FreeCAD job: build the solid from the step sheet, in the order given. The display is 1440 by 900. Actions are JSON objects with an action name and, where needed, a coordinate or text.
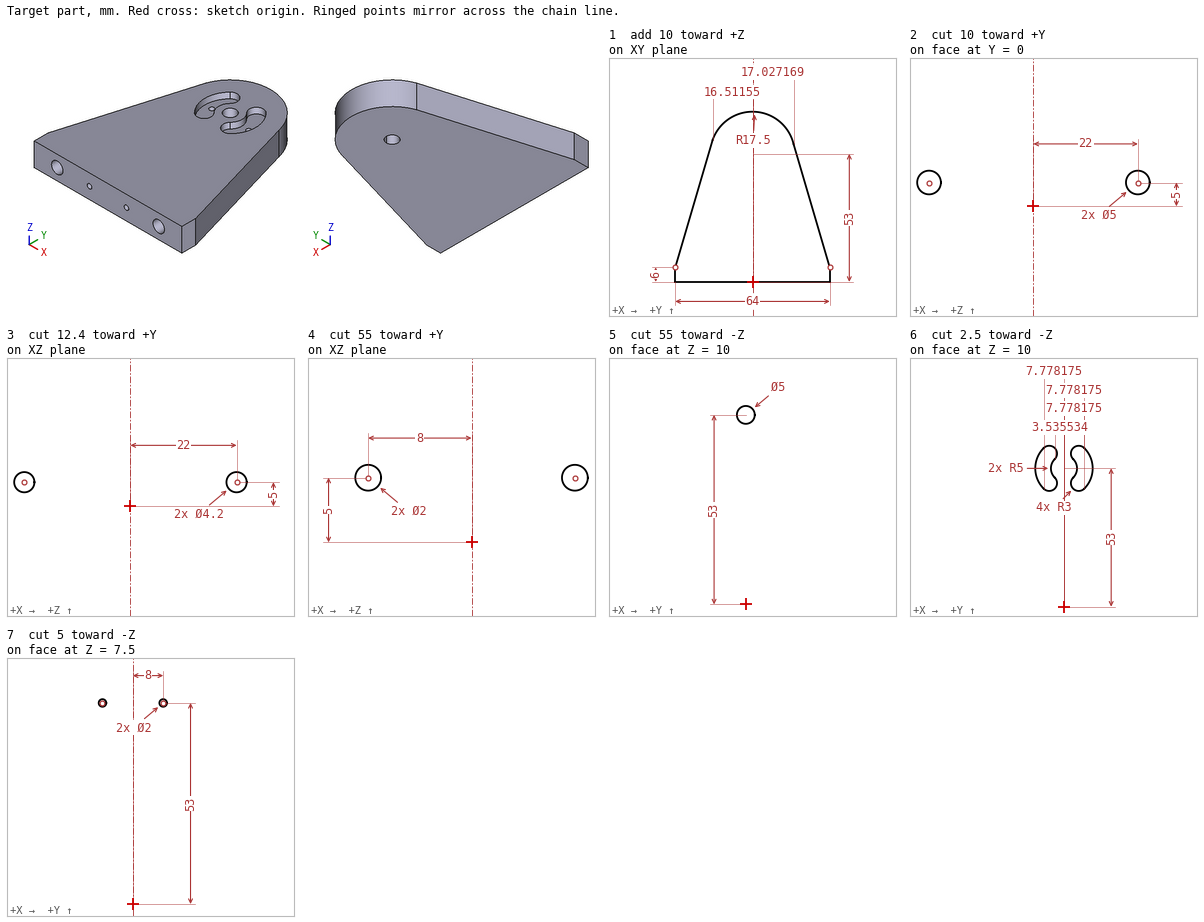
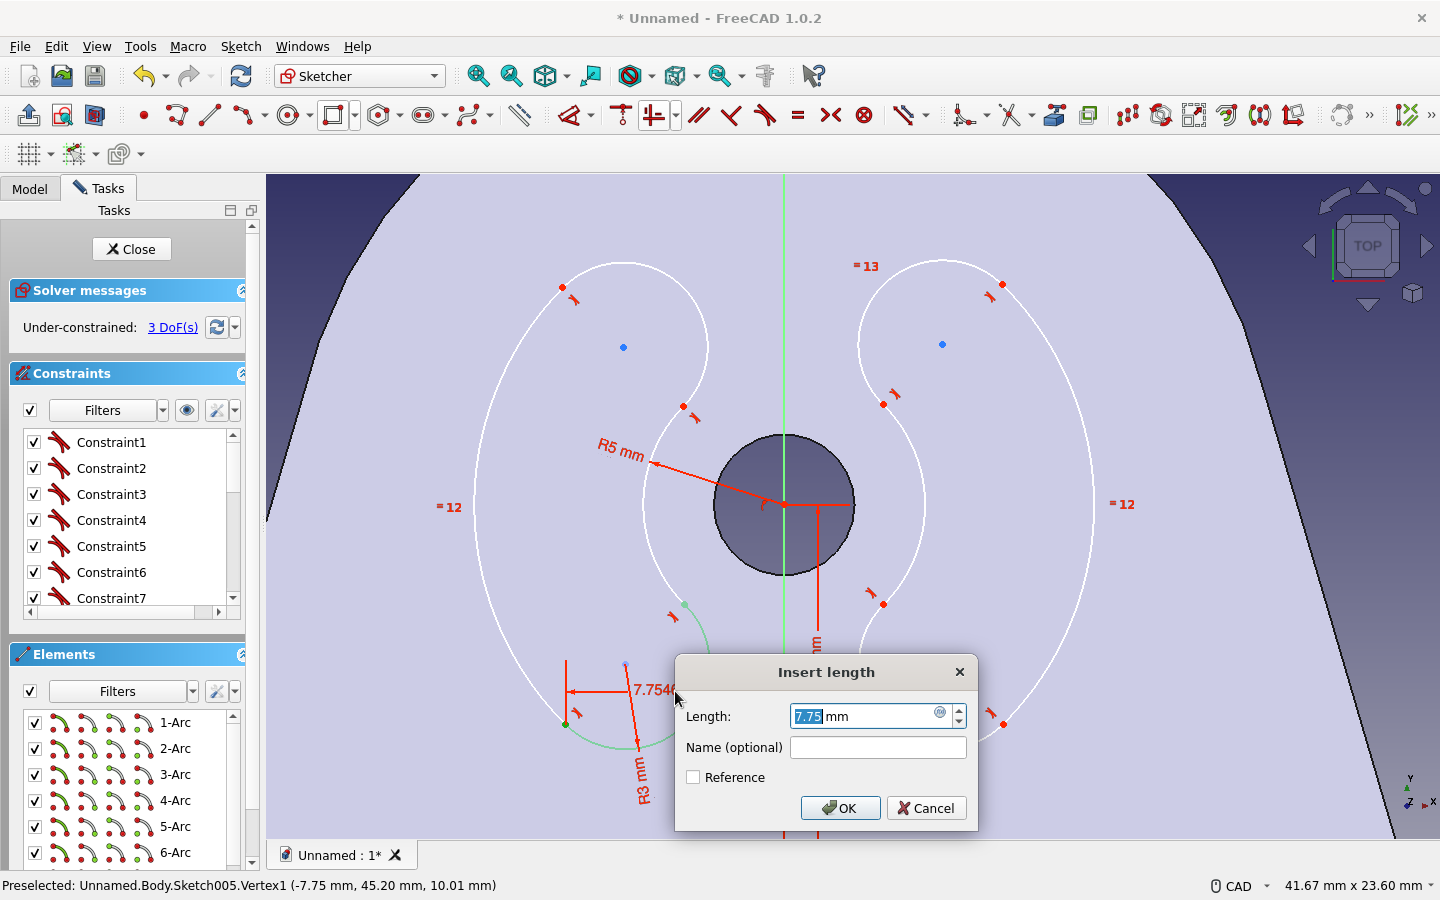
{"action": "type", "text": "7.778175"}
{"action": "key", "text": "Return"}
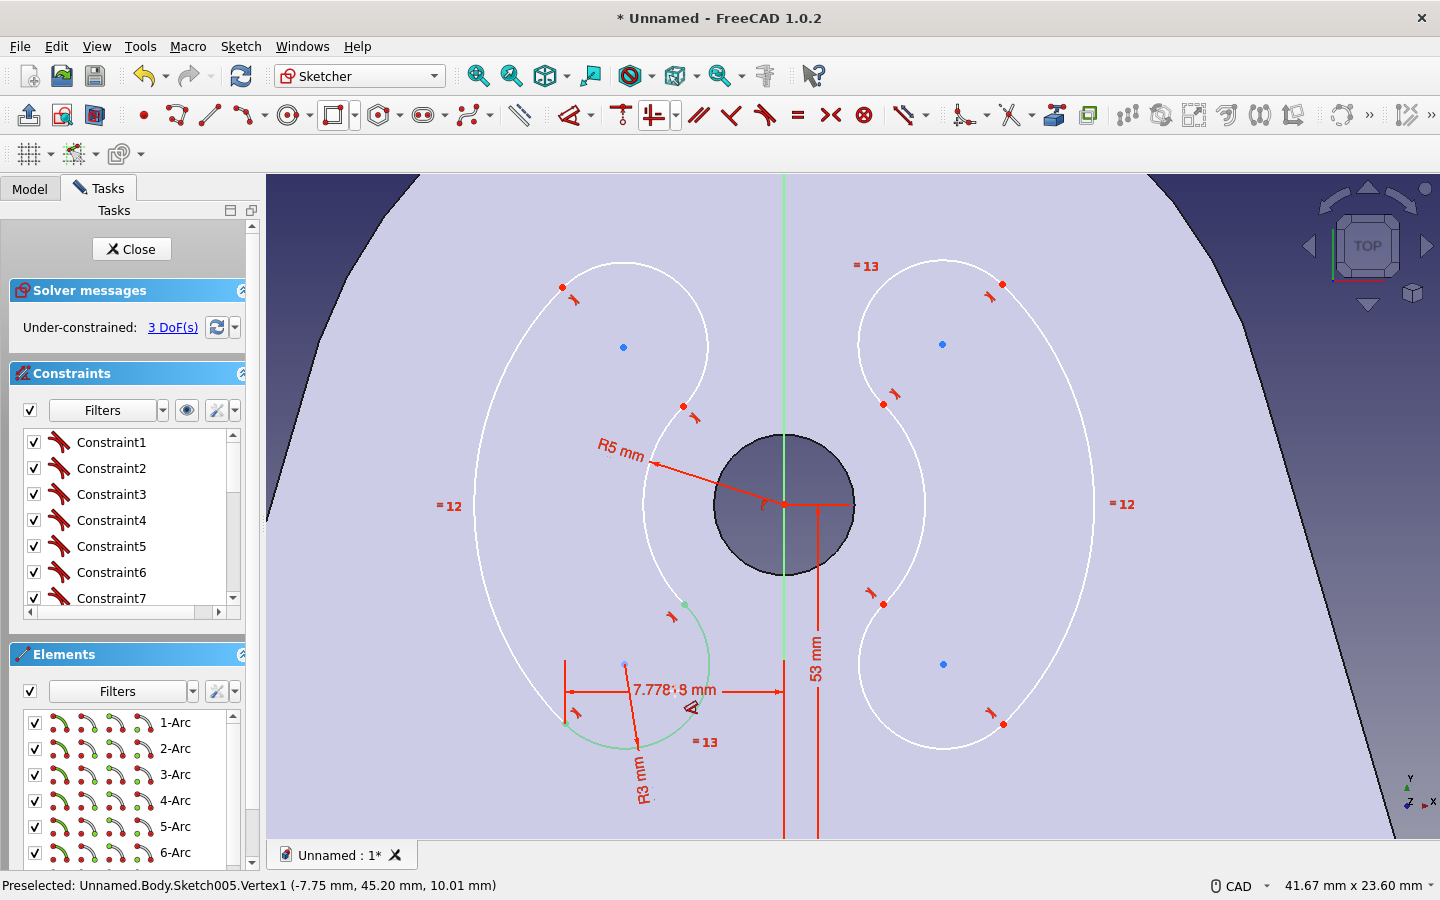
{"action": "left_click", "coordinate": [684, 406]}
{"action": "left_click", "coordinate": [734, 372]}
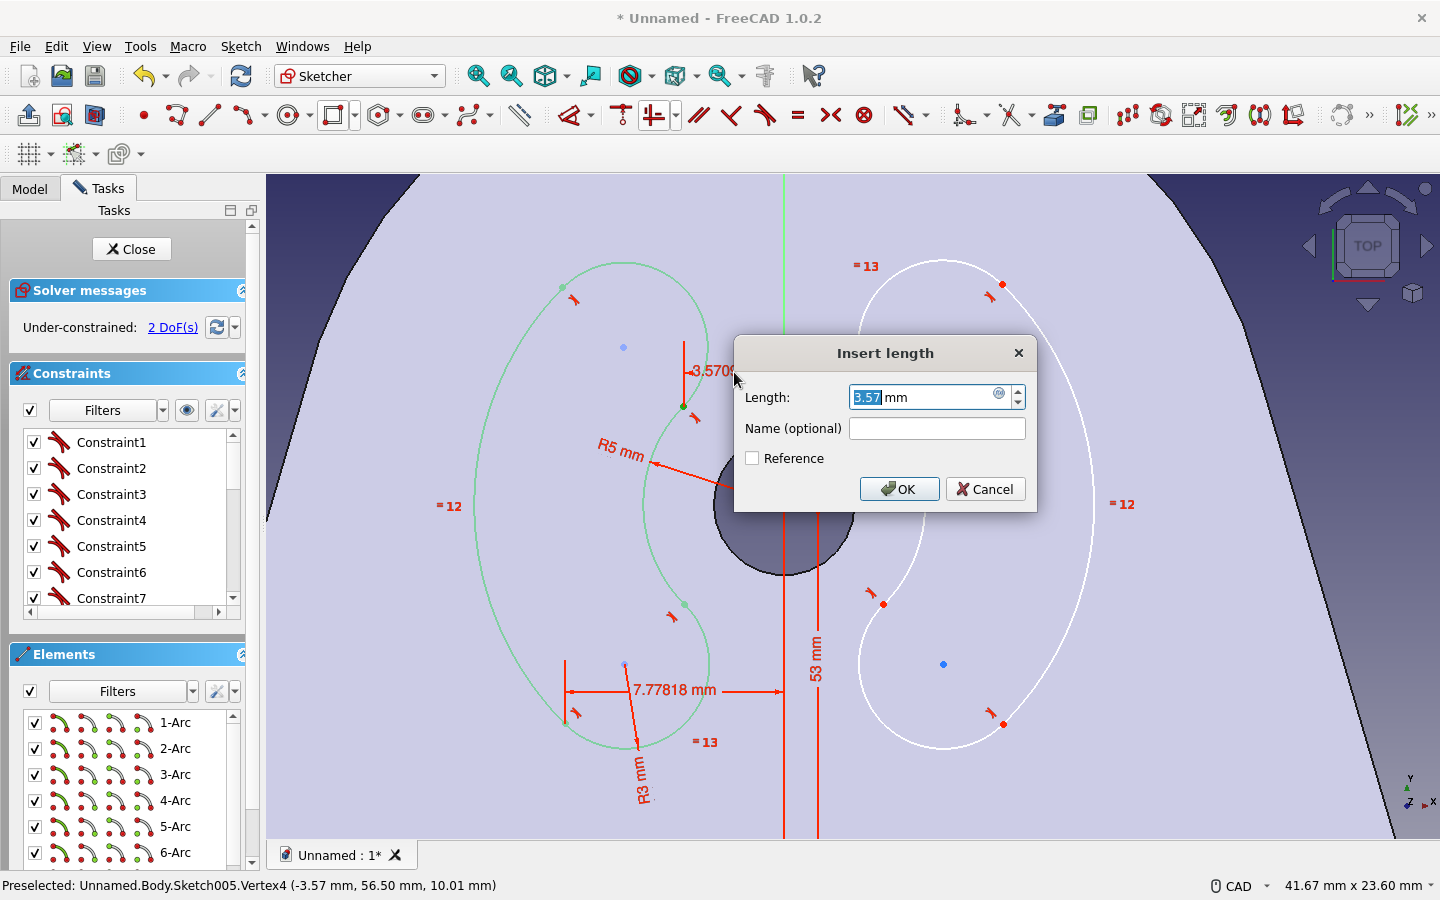
{"action": "type", "text": "3.535534"}
{"action": "key", "text": "Return"}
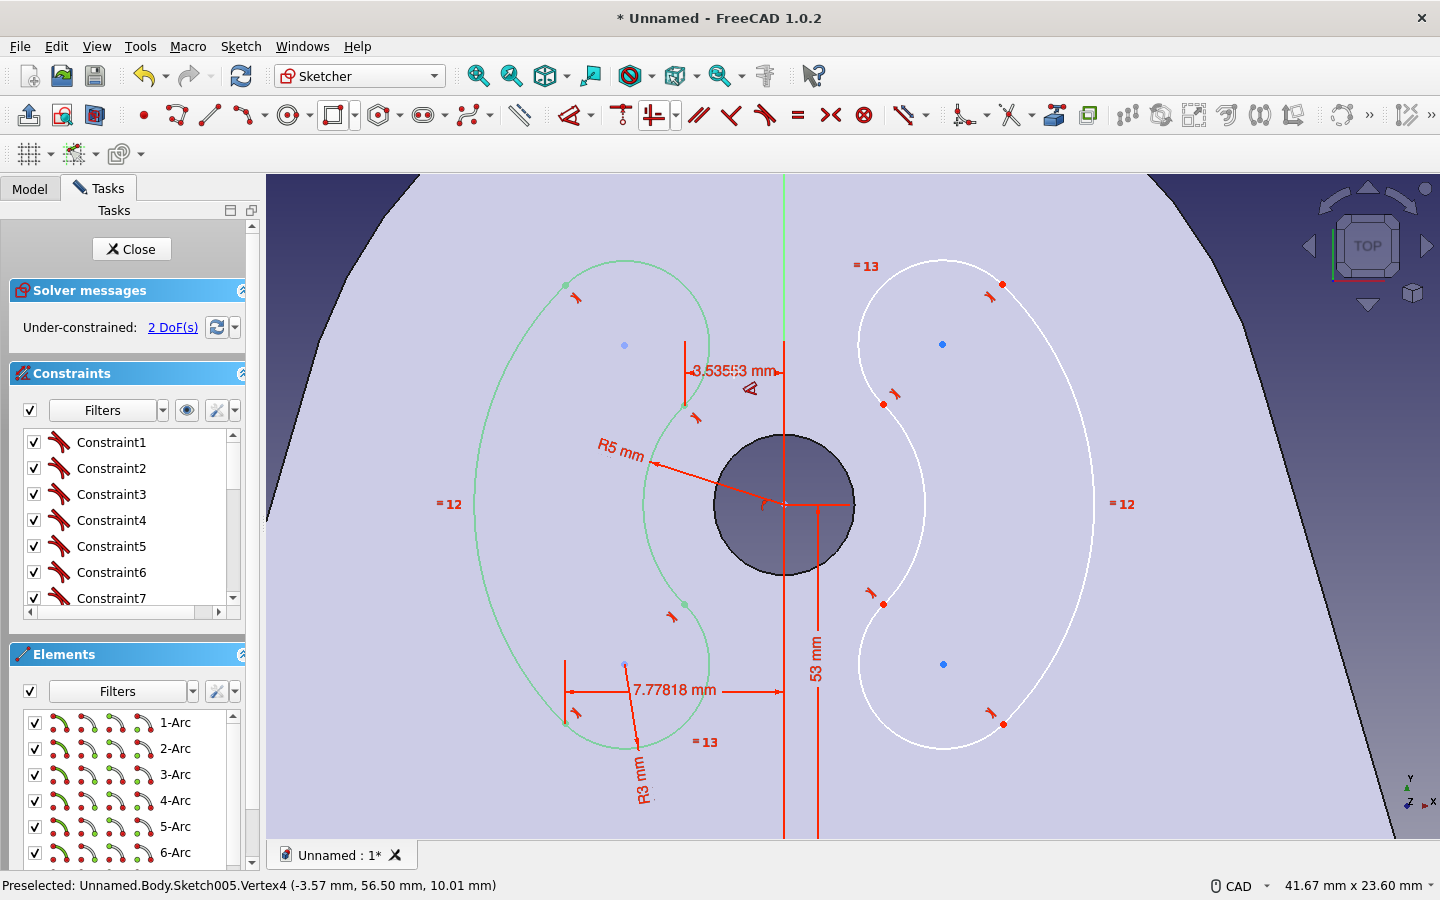
{"action": "left_click", "coordinate": [1003, 724]}
{"action": "left_click", "coordinate": [894, 690]}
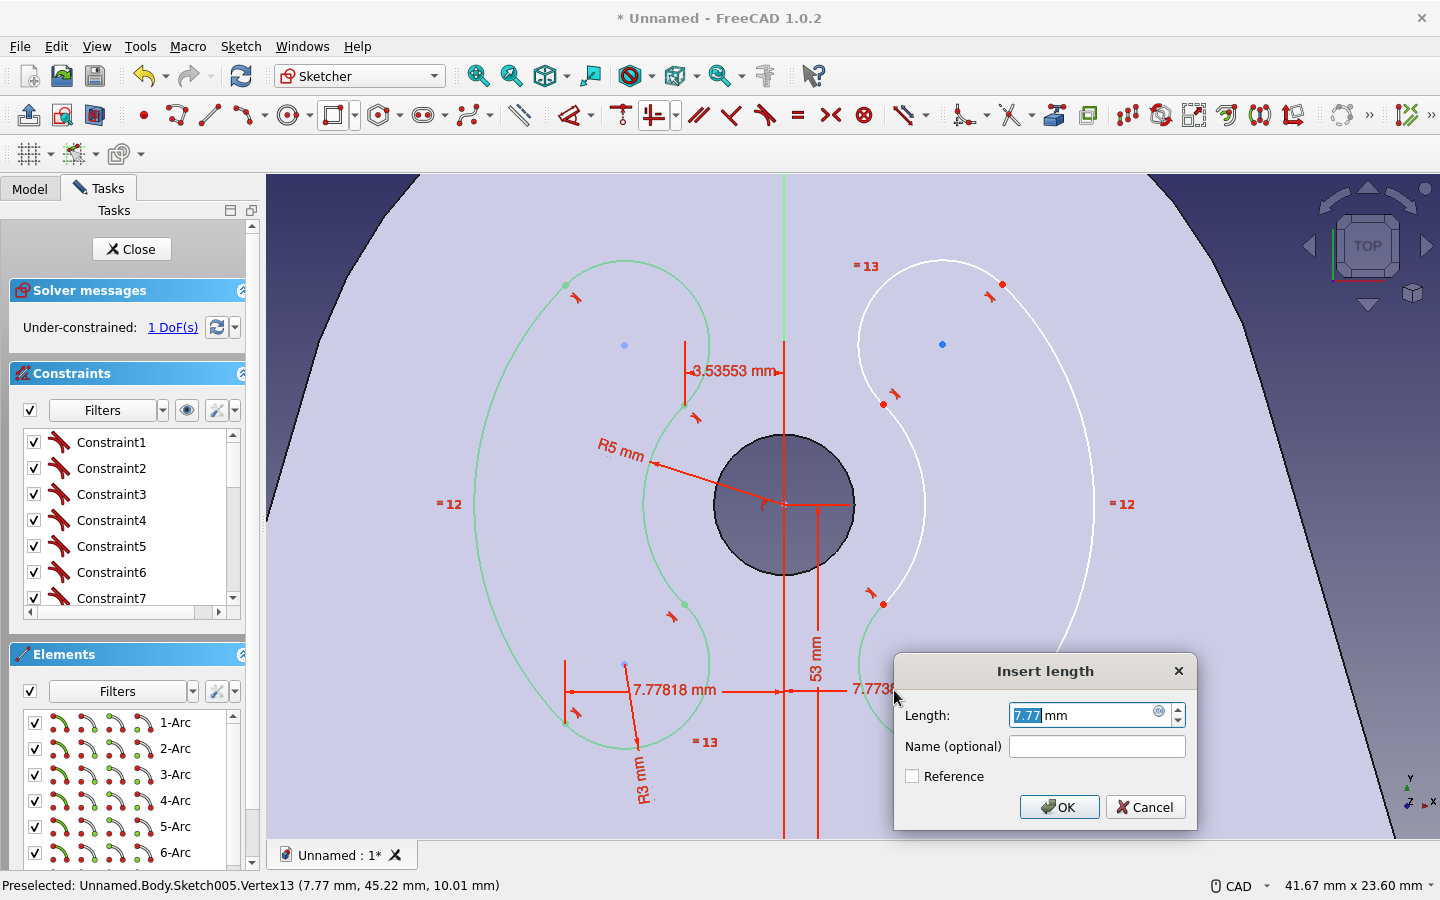
{"action": "type", "text": "7.778175"}
{"action": "key", "text": "Return"}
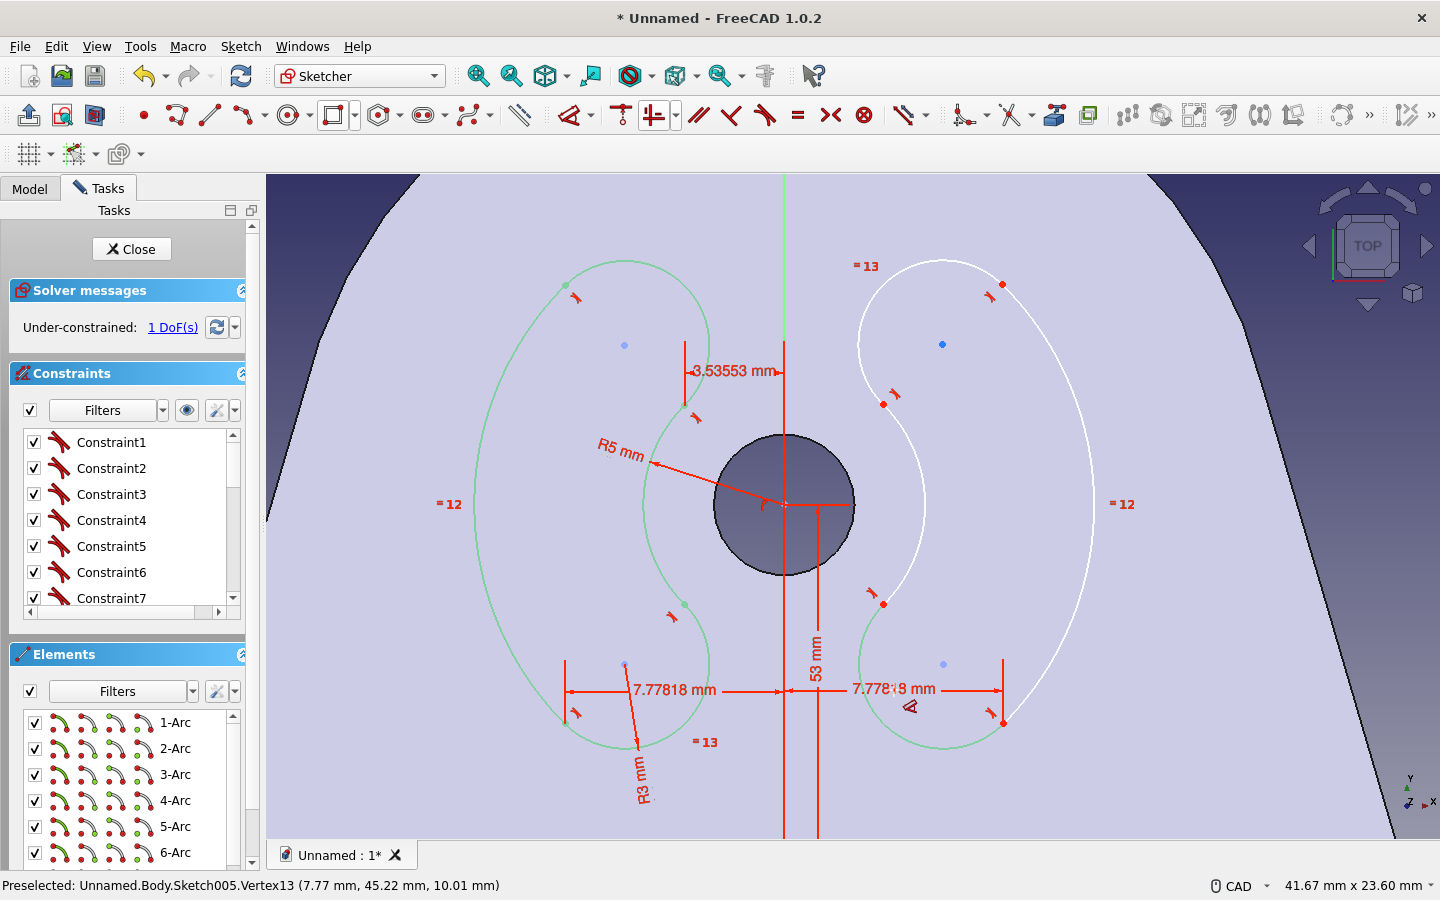
{"action": "left_click", "coordinate": [1002, 285]}
{"action": "left_click", "coordinate": [893, 251]}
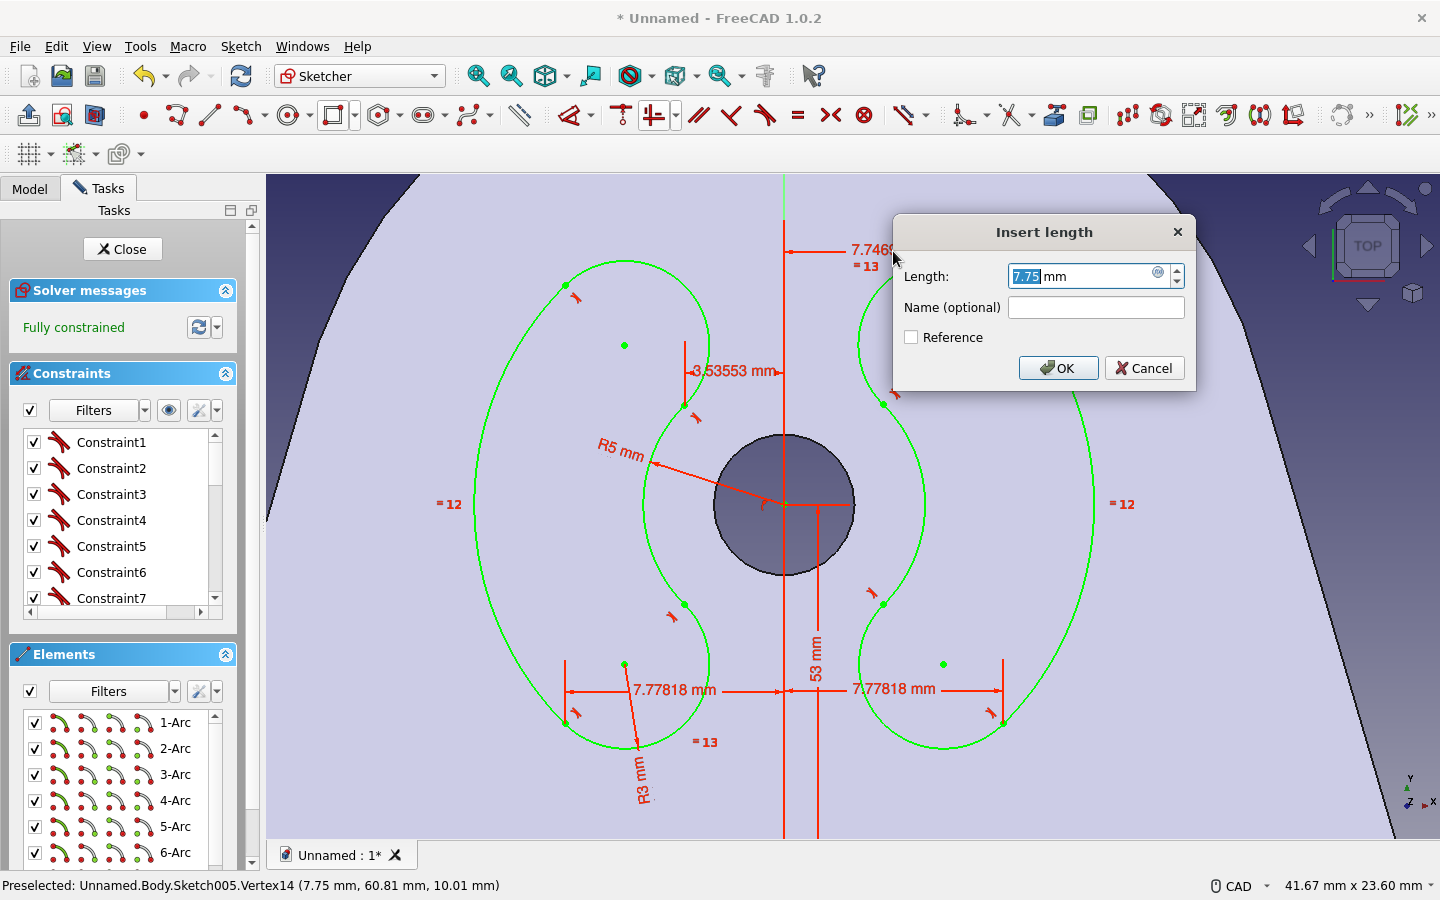
{"action": "type", "text": "7.778175"}
{"action": "key", "text": "Return"}
{"action": "key", "text": "Escape"}